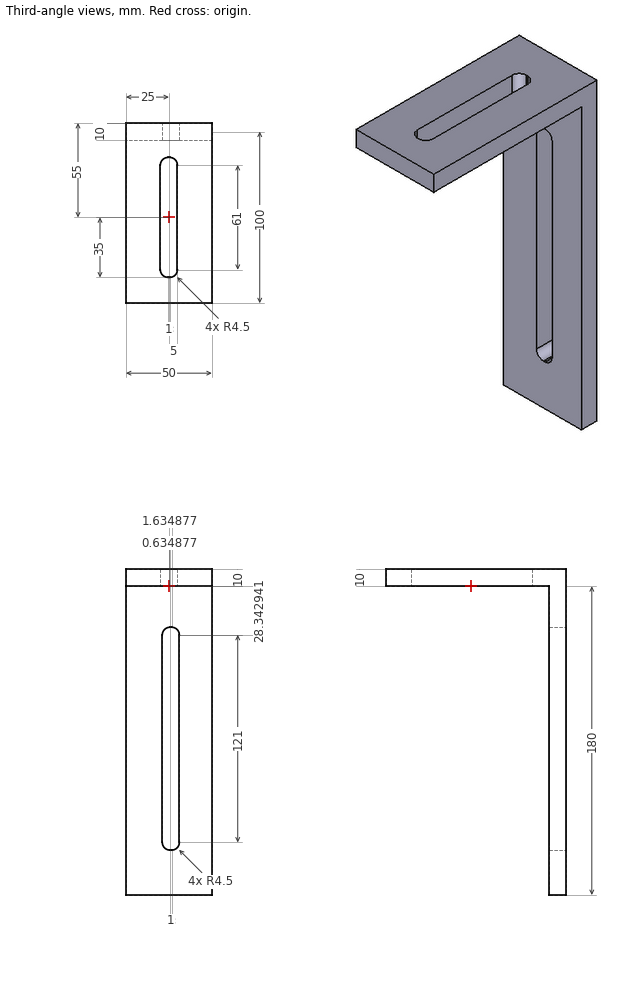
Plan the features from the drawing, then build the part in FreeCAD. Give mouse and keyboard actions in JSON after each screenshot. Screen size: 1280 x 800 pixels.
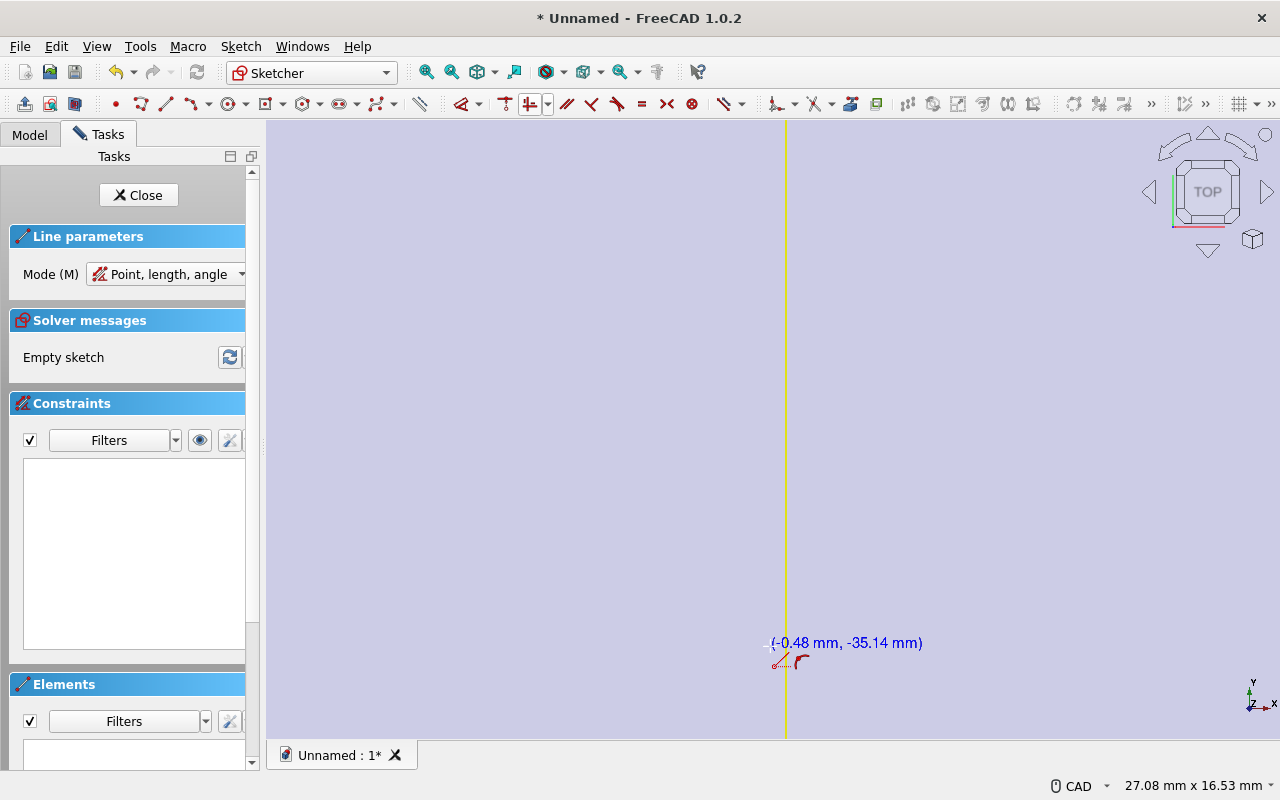
{"action": "left_click", "coordinate": [767, 643]}
{"action": "left_click", "coordinate": [804, 643]}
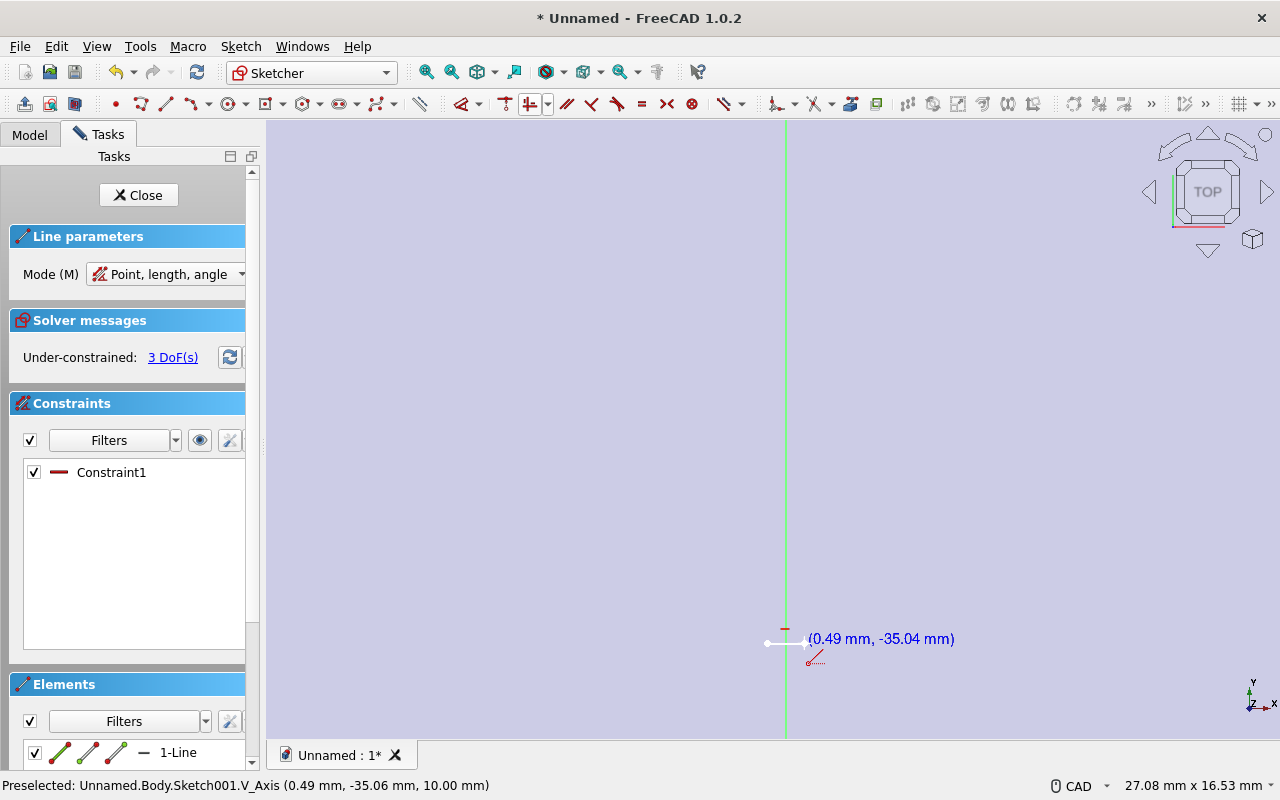
{"action": "scroll", "coordinate": [688, 647], "scroll_direction": "down", "scroll_amount": 9}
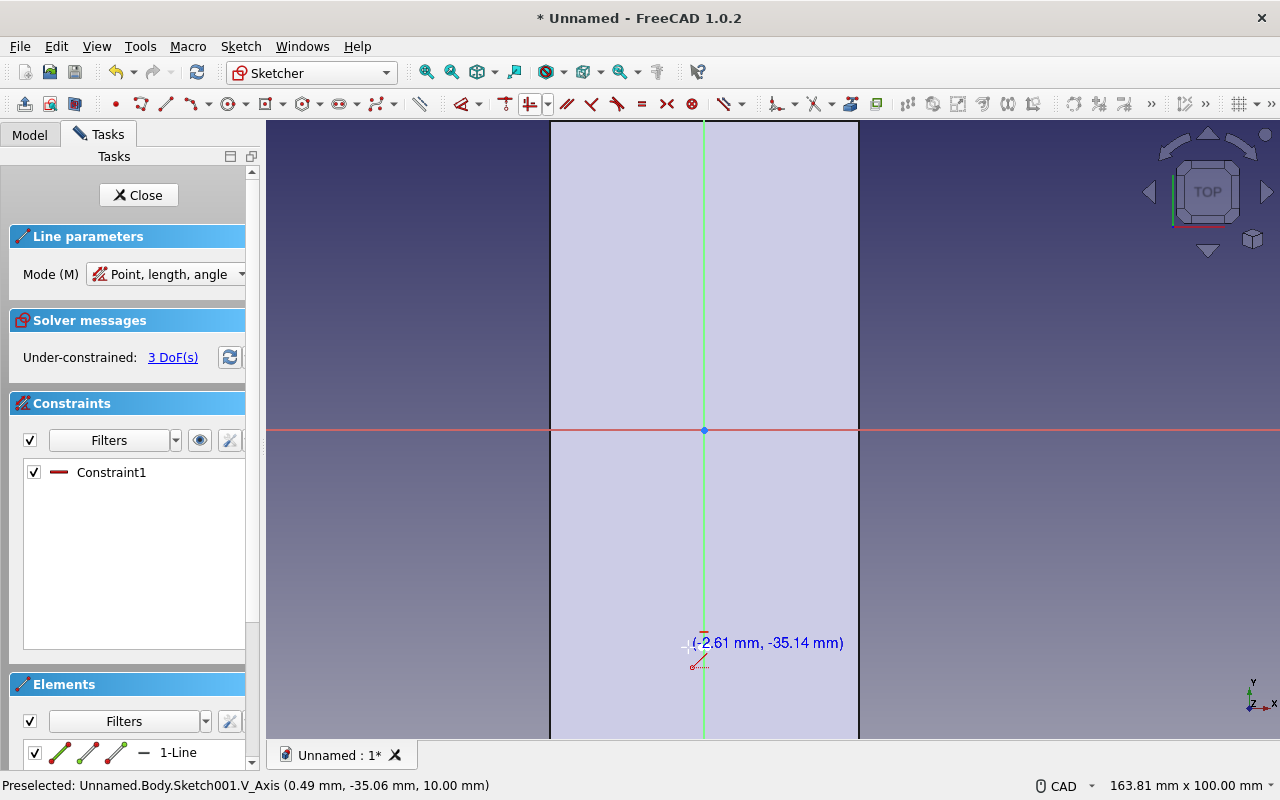
{"action": "left_click", "coordinate": [735, 619]}
{"action": "left_click", "coordinate": [735, 242]}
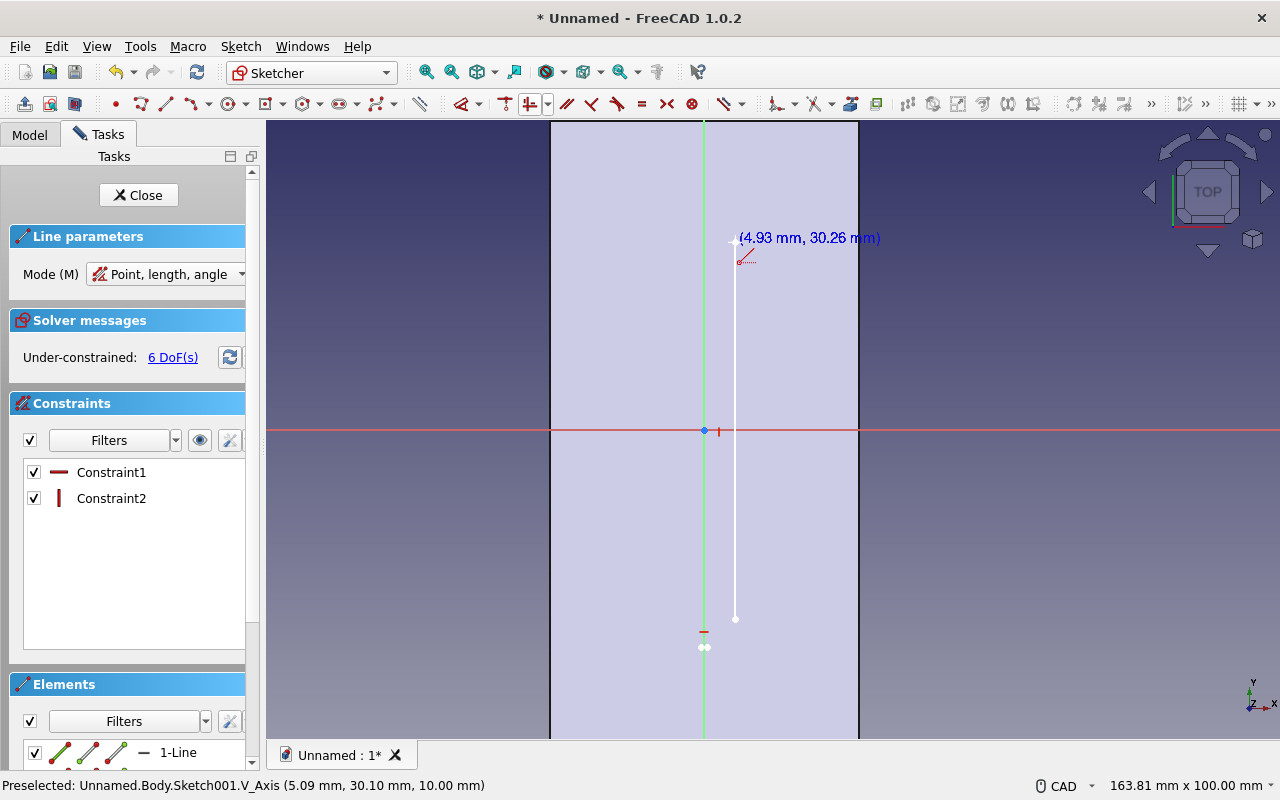
{"action": "scroll", "coordinate": [708, 214], "scroll_direction": "up", "scroll_amount": 9}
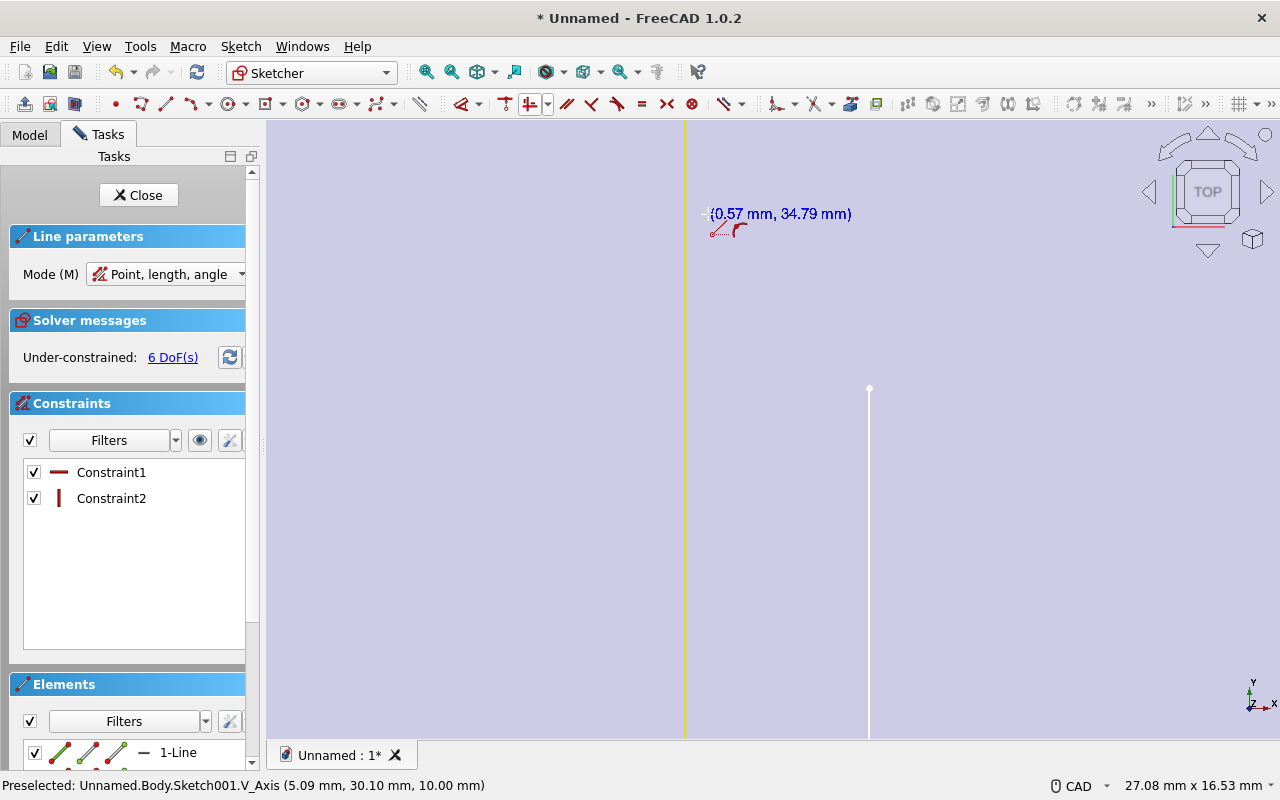
{"action": "left_click", "coordinate": [703, 211]}
{"action": "left_click", "coordinate": [666, 211]}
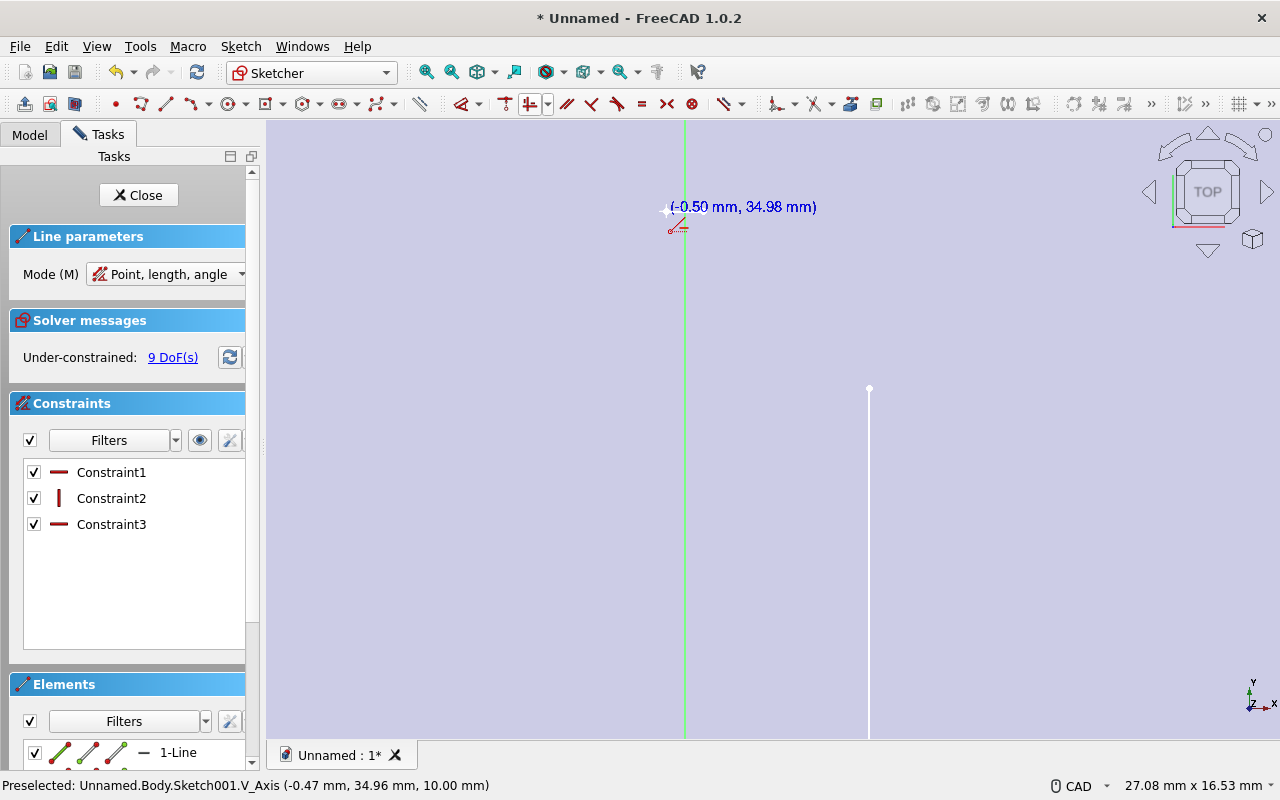
{"action": "scroll", "coordinate": [708, 213], "scroll_direction": "down", "scroll_amount": 9}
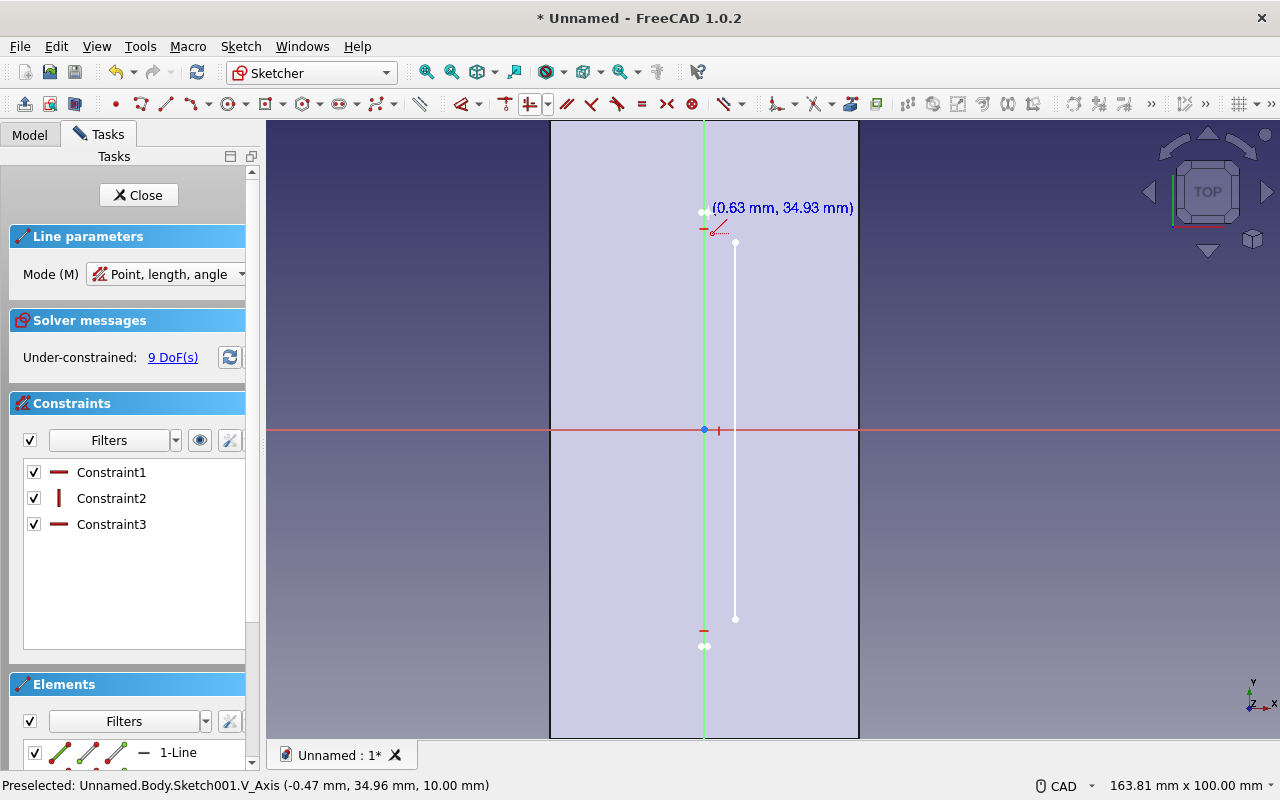
{"action": "left_click", "coordinate": [674, 241]}
{"action": "left_click", "coordinate": [674, 618]}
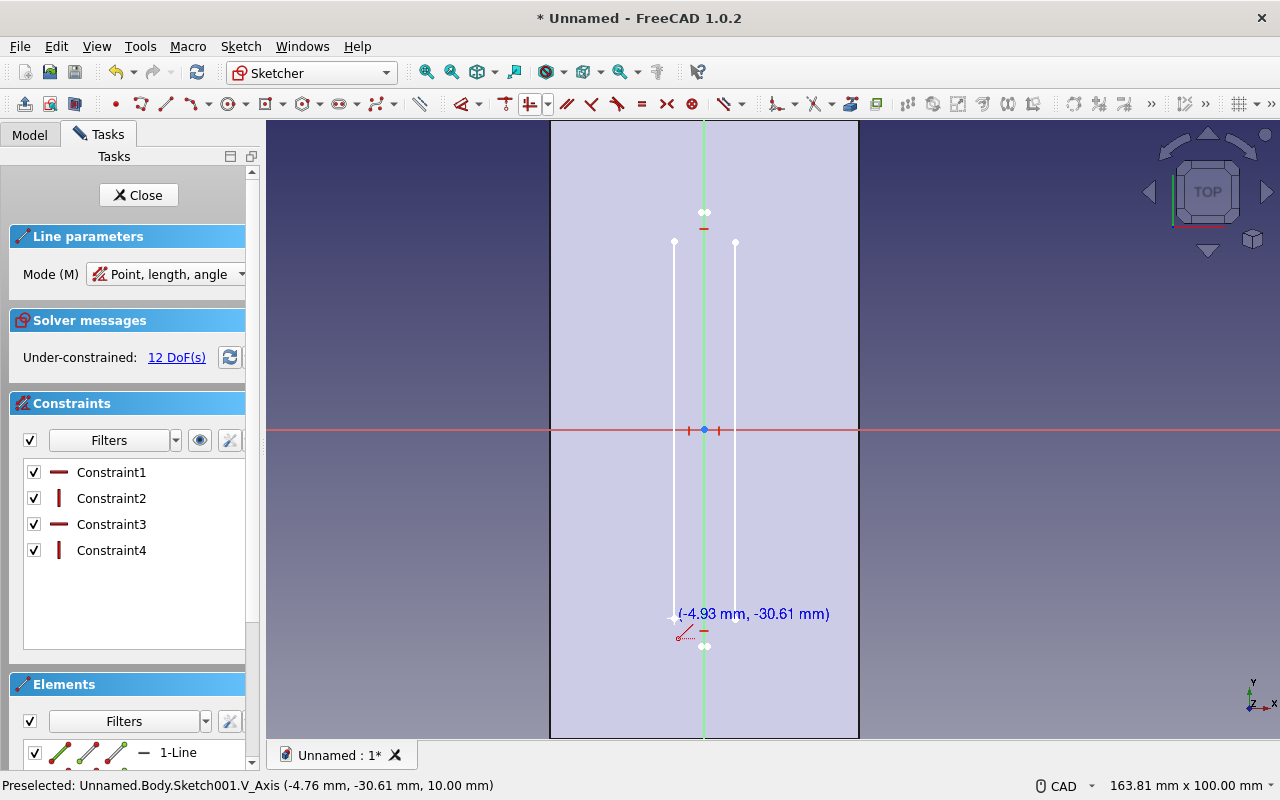
{"action": "left_click", "coordinate": [190, 104]}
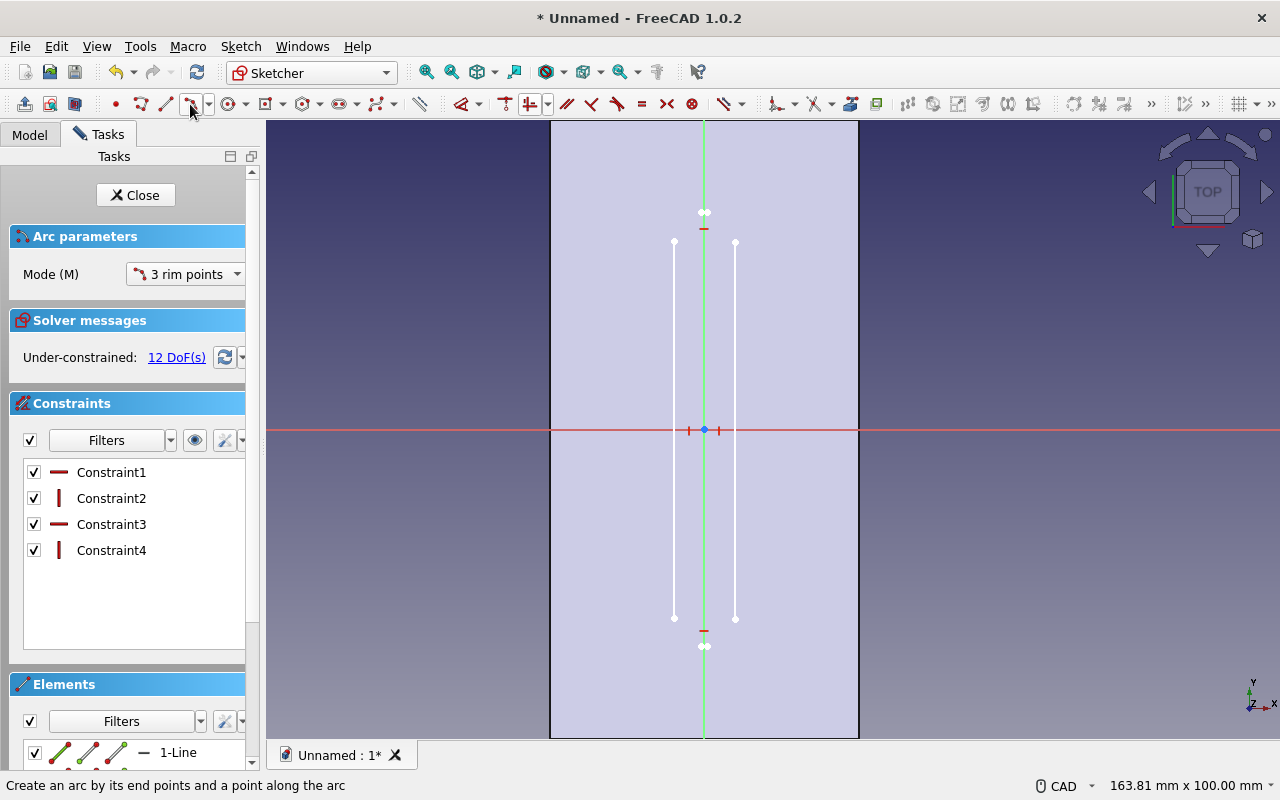
{"action": "scroll", "coordinate": [708, 646], "scroll_direction": "up", "scroll_amount": 9}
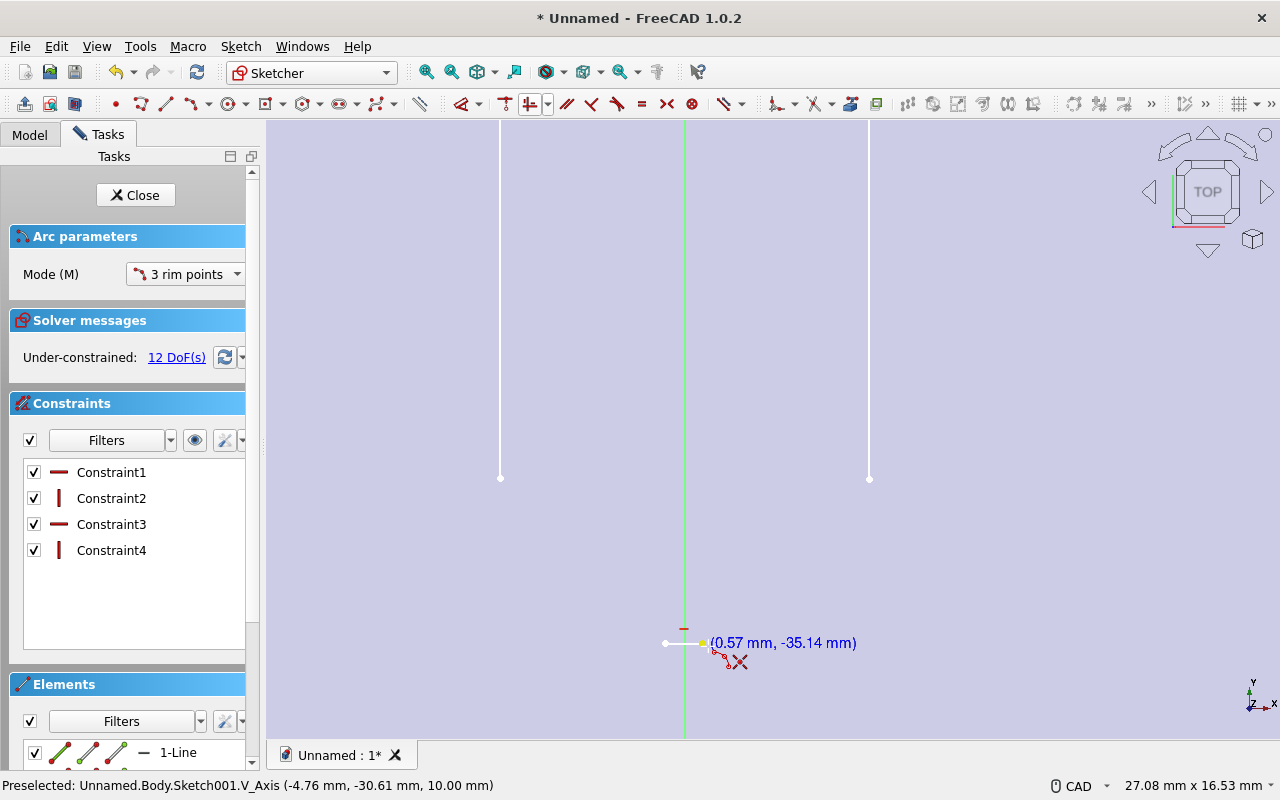
{"action": "left_click", "coordinate": [703, 644]}